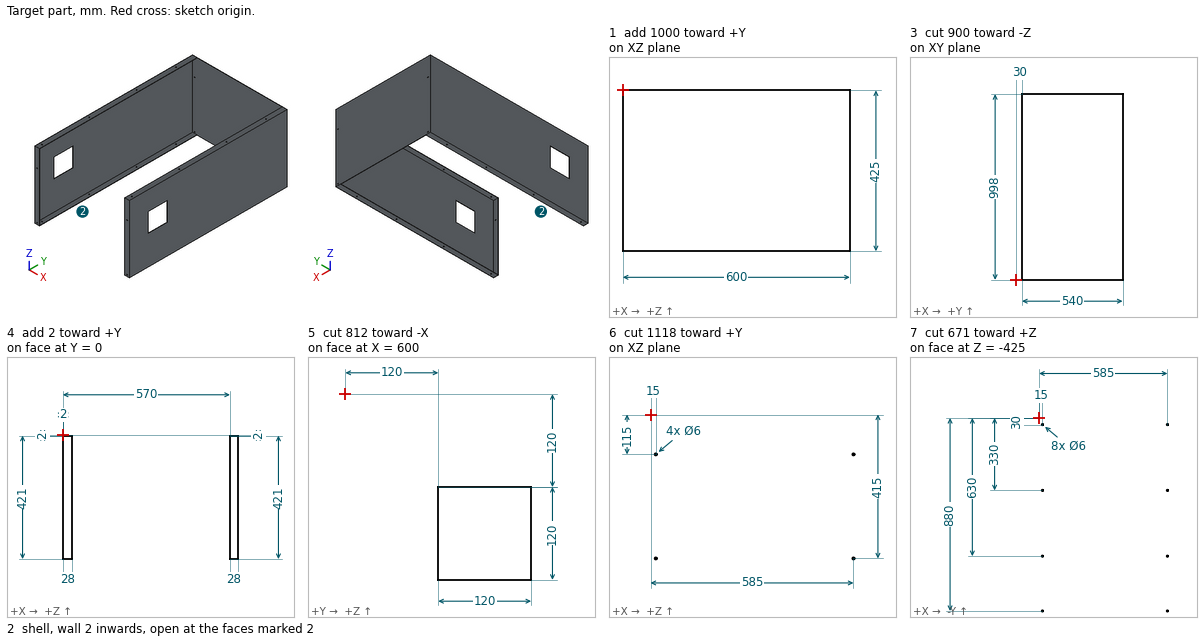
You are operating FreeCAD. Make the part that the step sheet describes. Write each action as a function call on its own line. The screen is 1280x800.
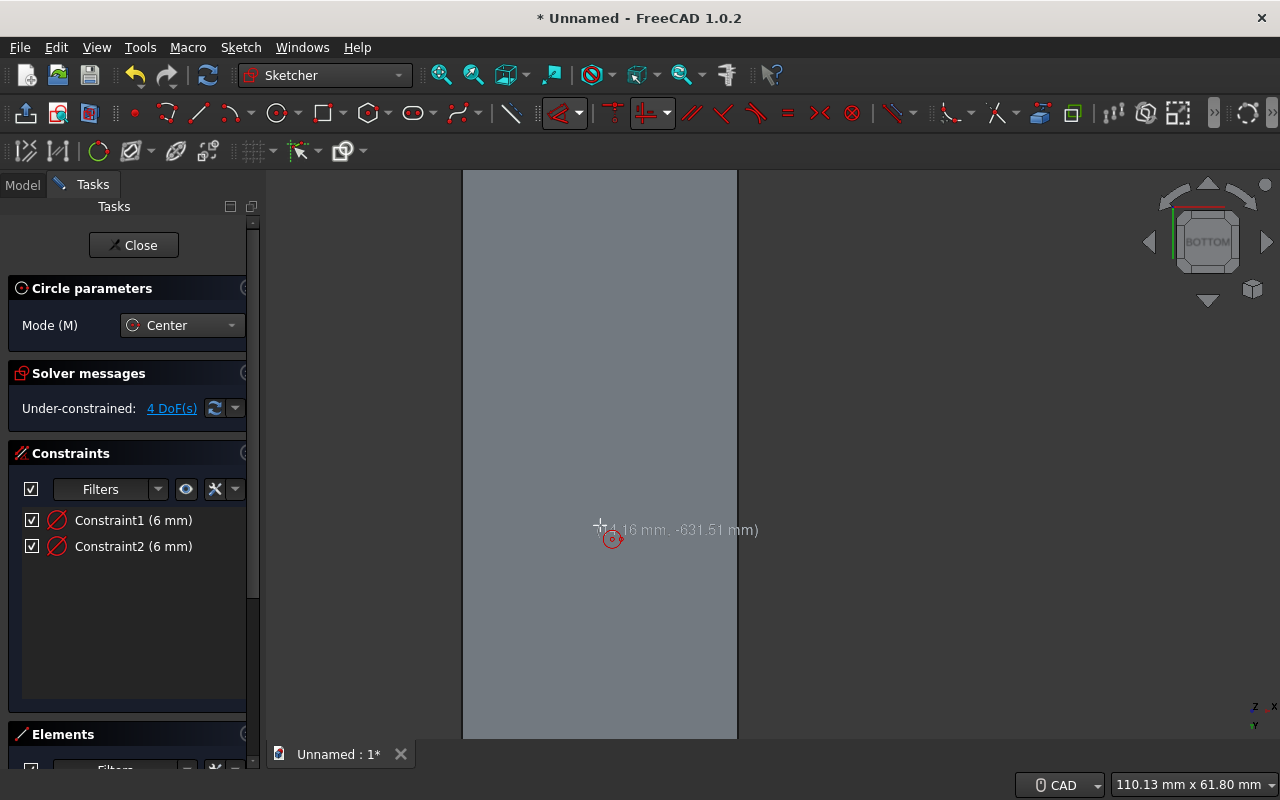
scroll(575, 542, down, 15)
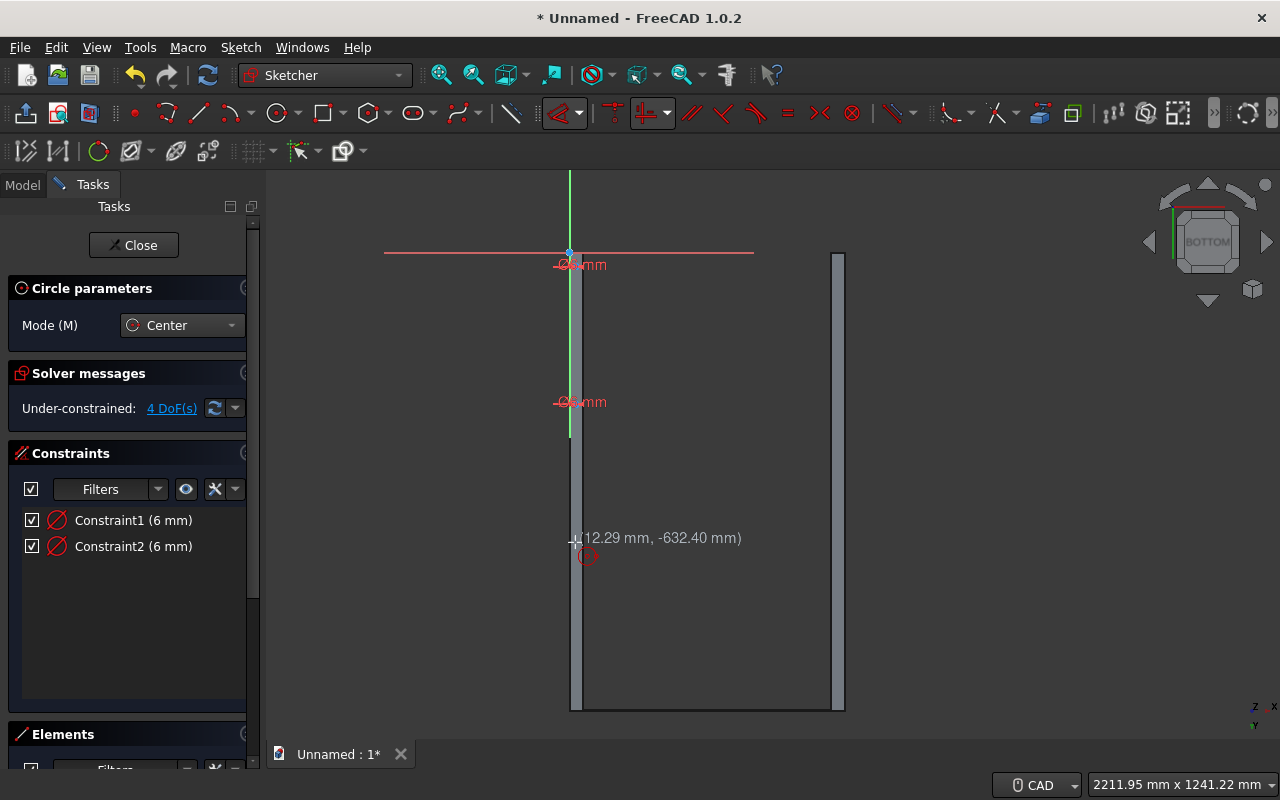
scroll(577, 542, up, 5)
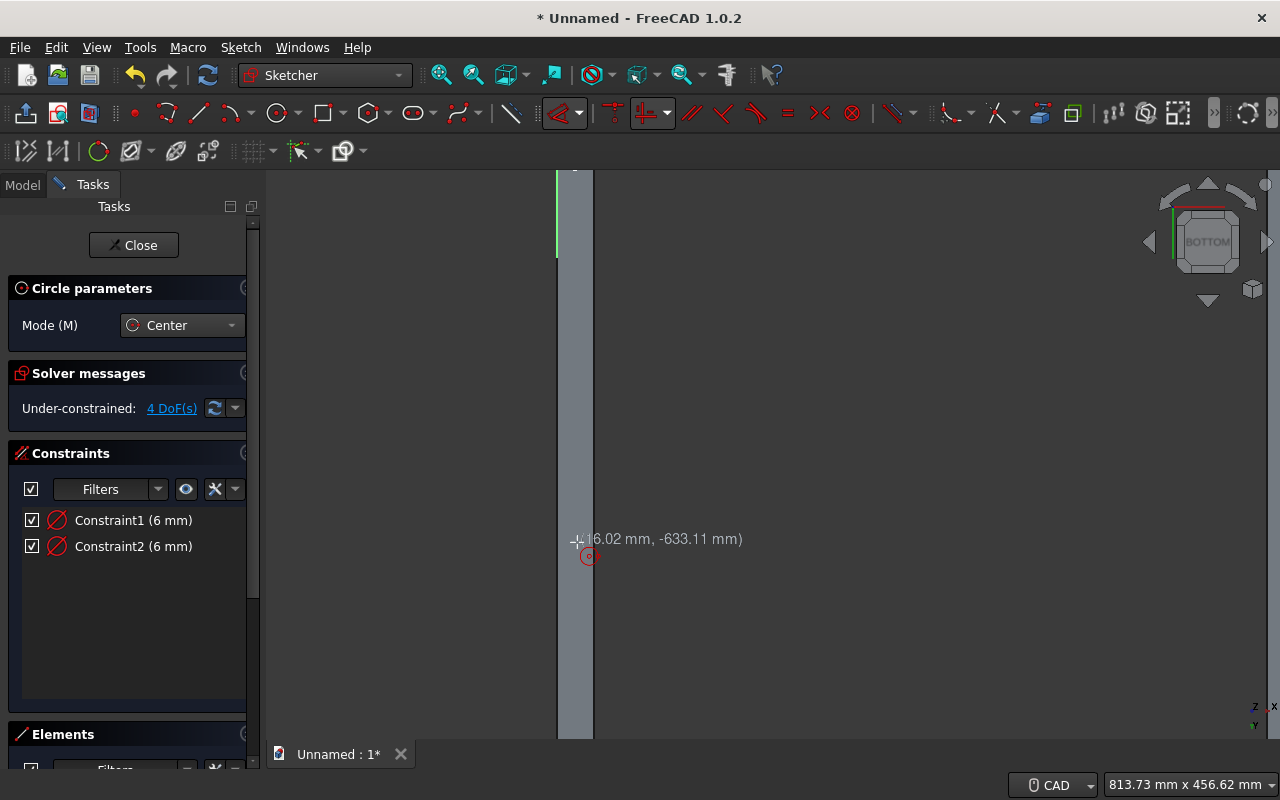
click(575, 540)
move(578, 537)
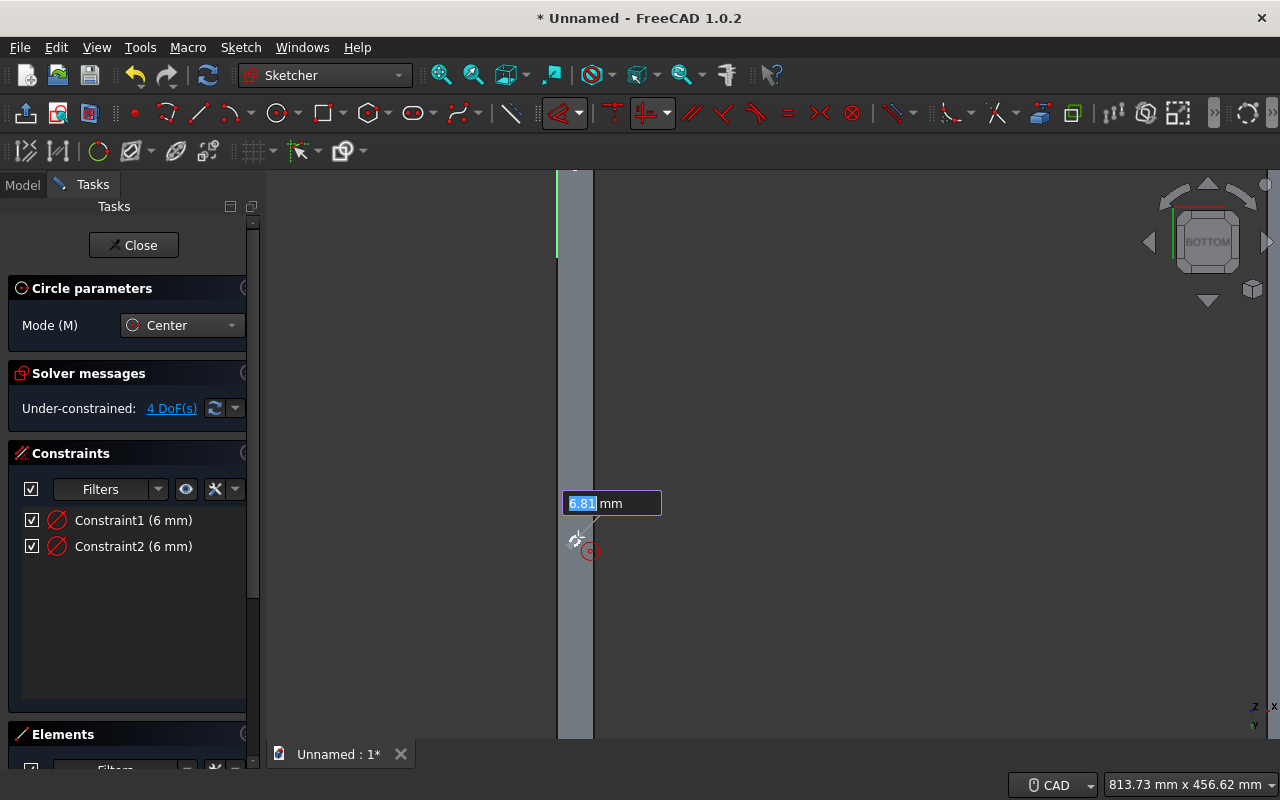
text(6)
key(Return)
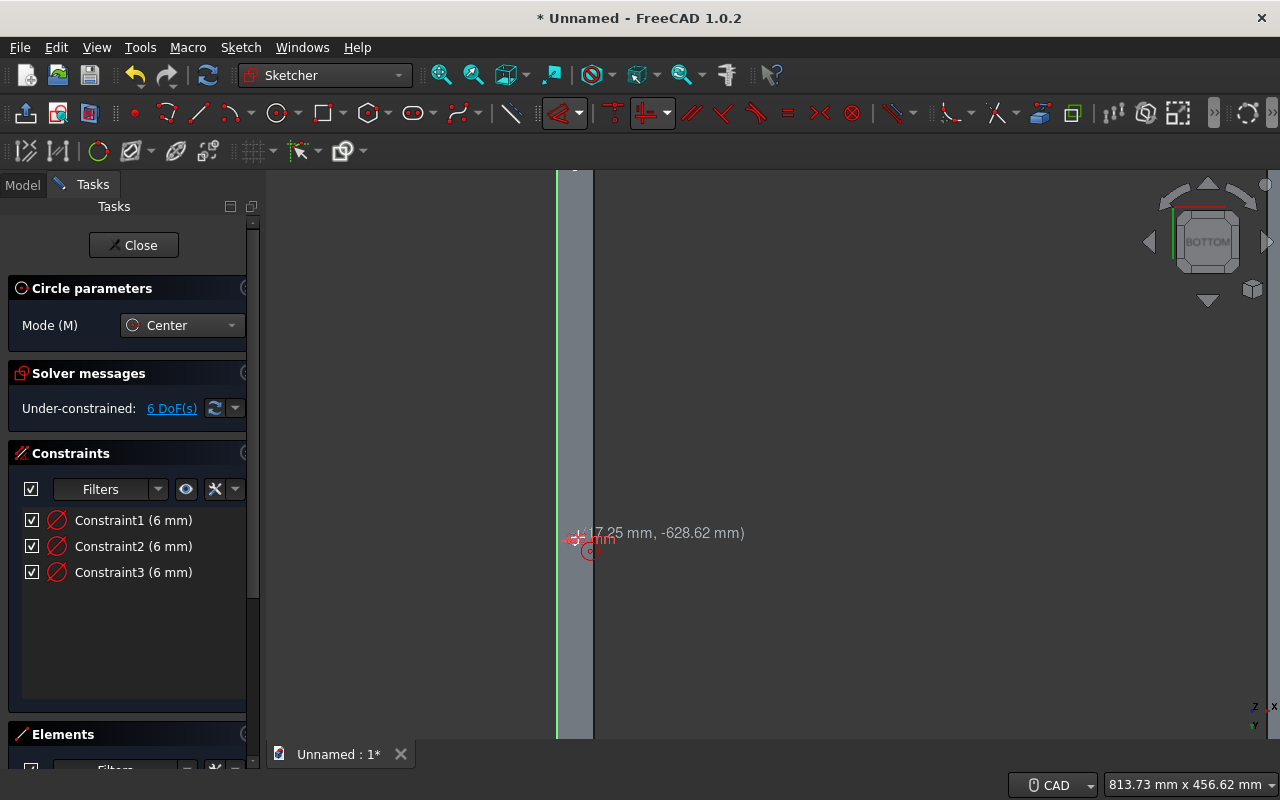
scroll(610, 519, down, 6)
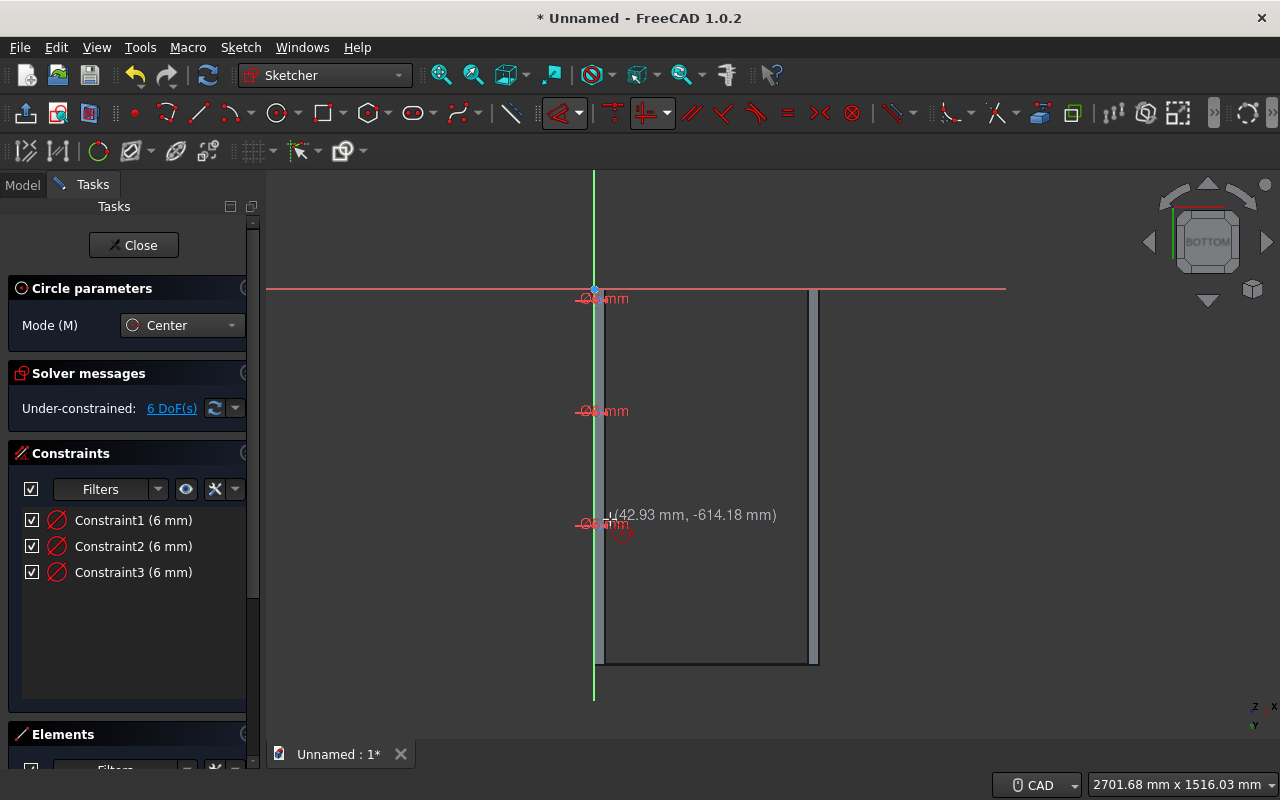
scroll(814, 300, up, 16)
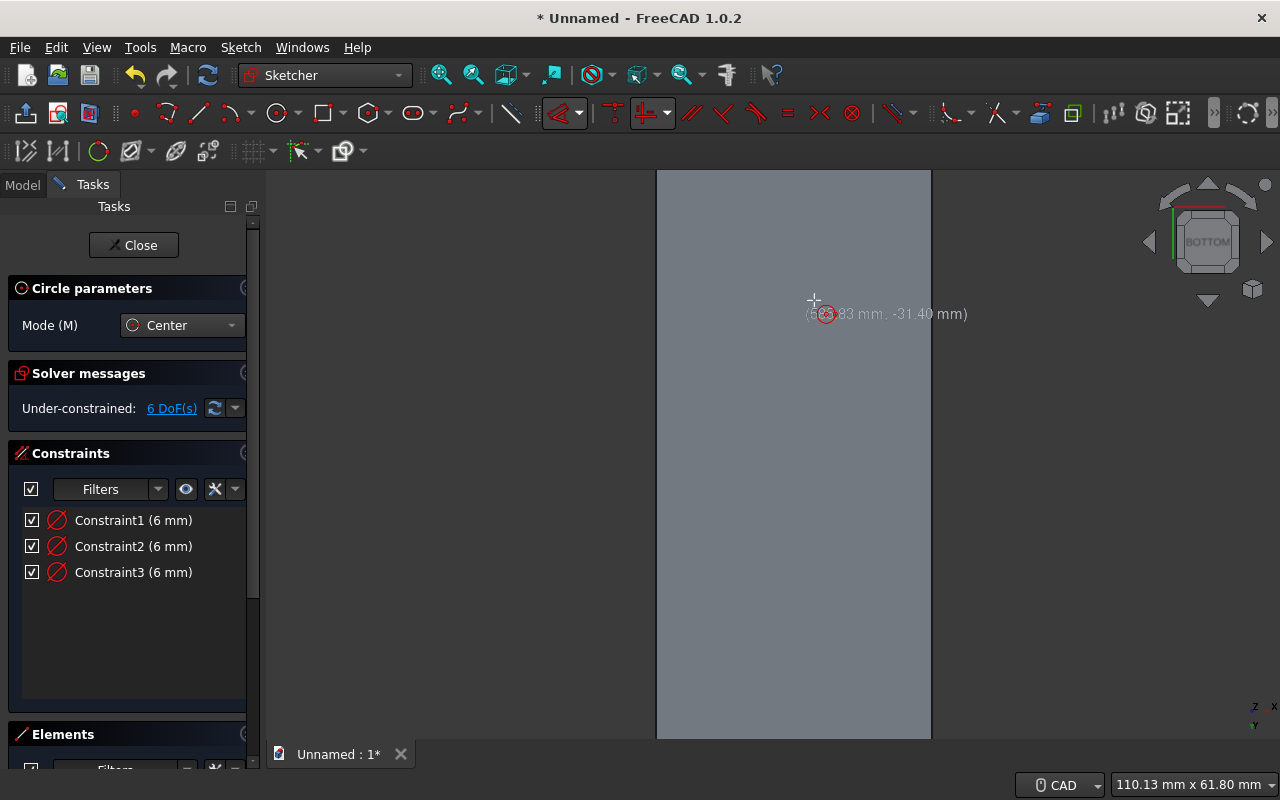
scroll(840, 264, down, 15)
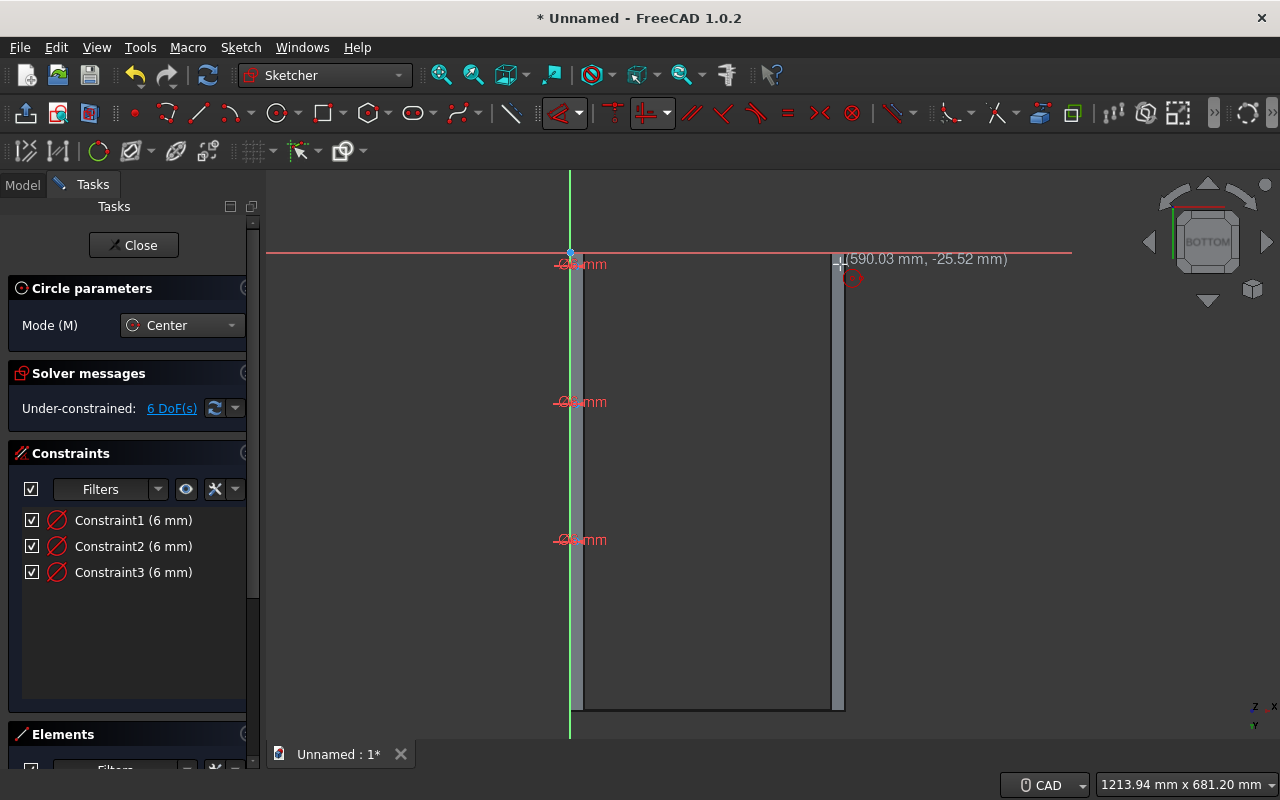
click(838, 266)
move(839, 267)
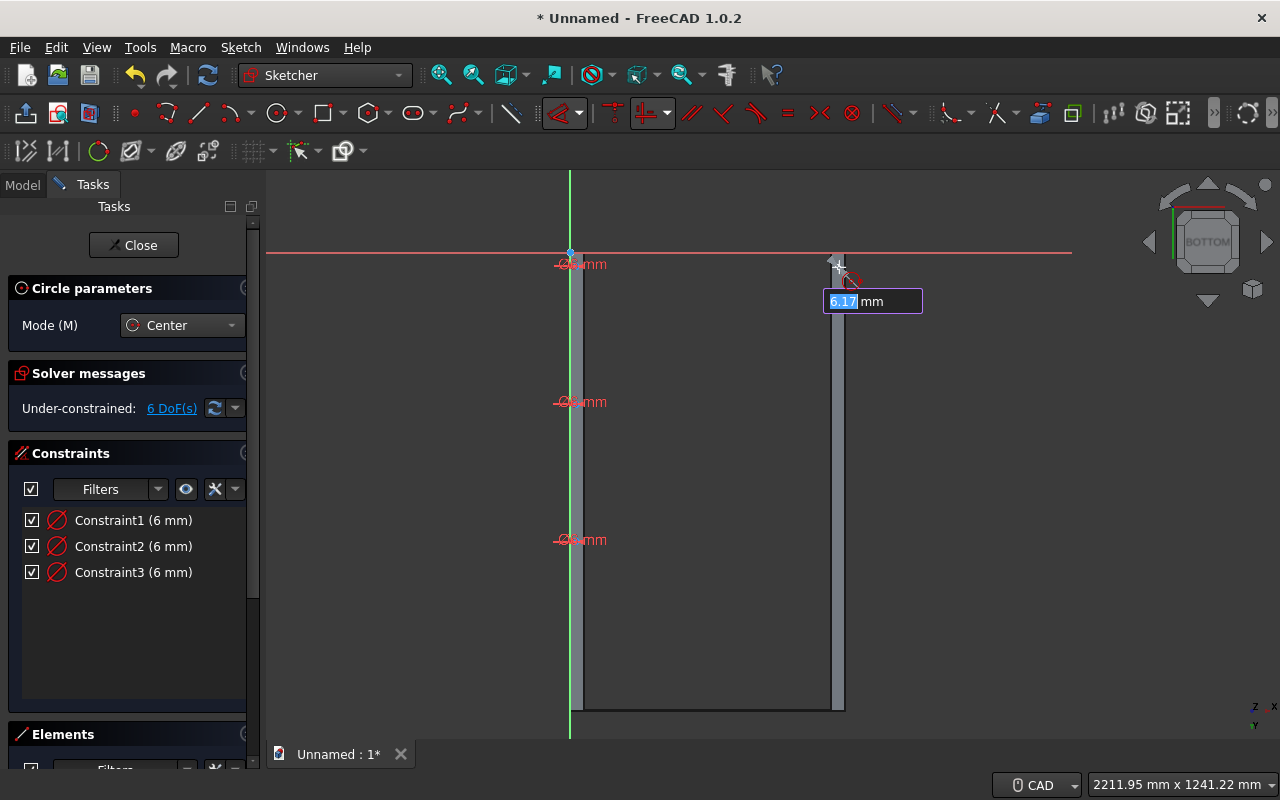
text(6)
key(Return)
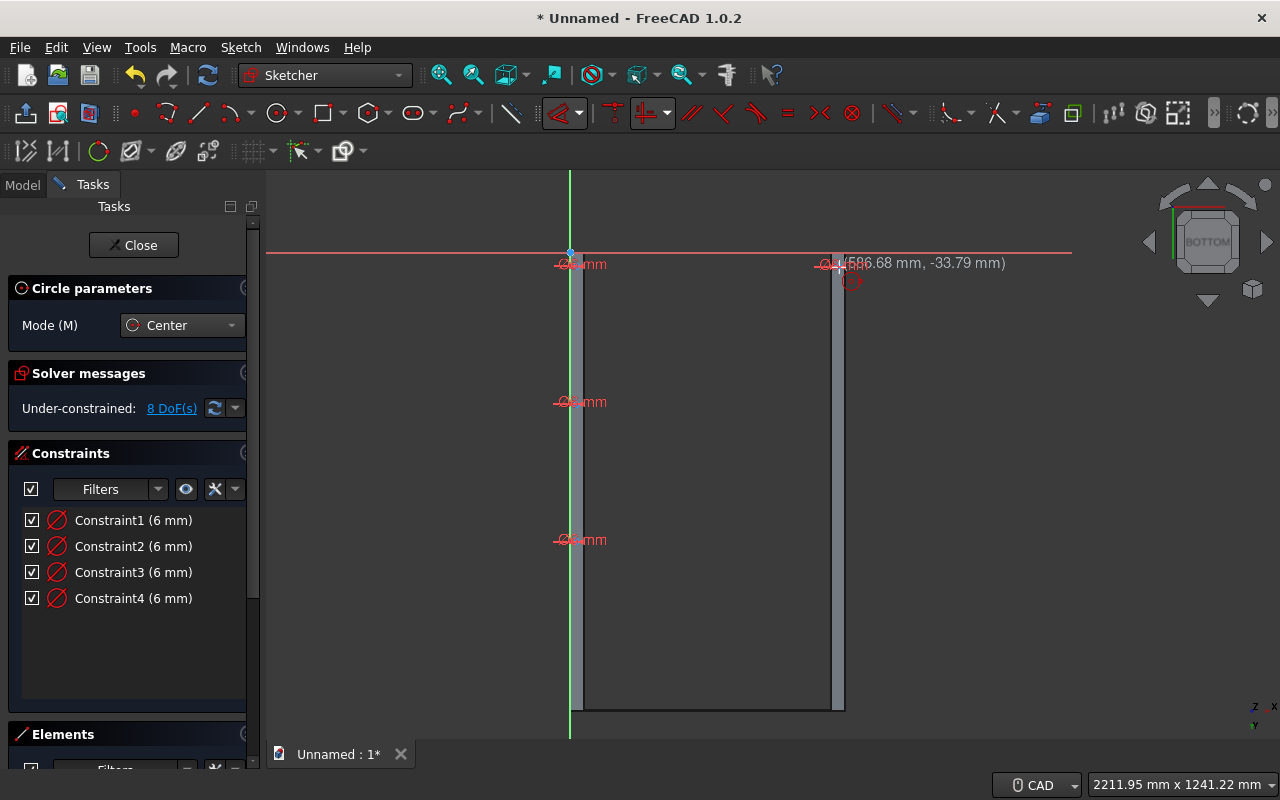
scroll(838, 404, up, 15)